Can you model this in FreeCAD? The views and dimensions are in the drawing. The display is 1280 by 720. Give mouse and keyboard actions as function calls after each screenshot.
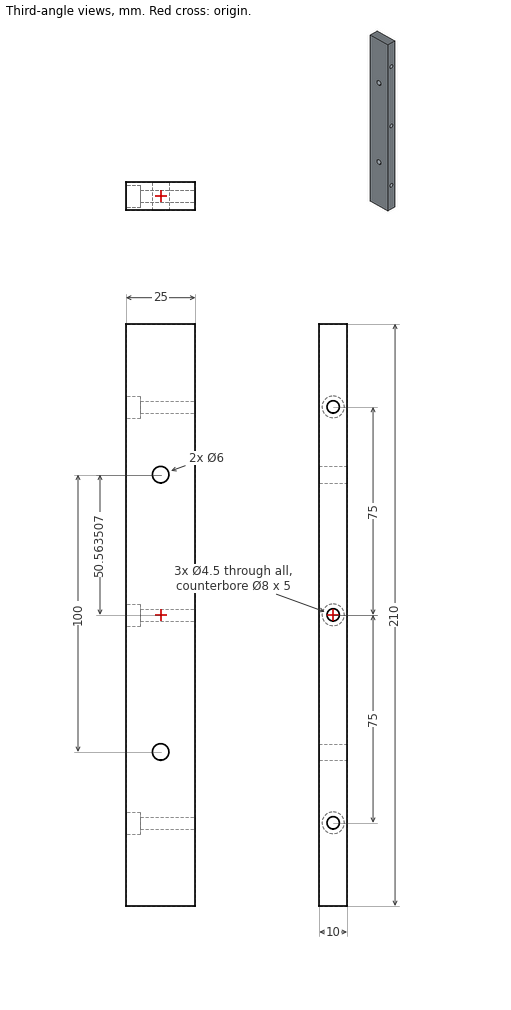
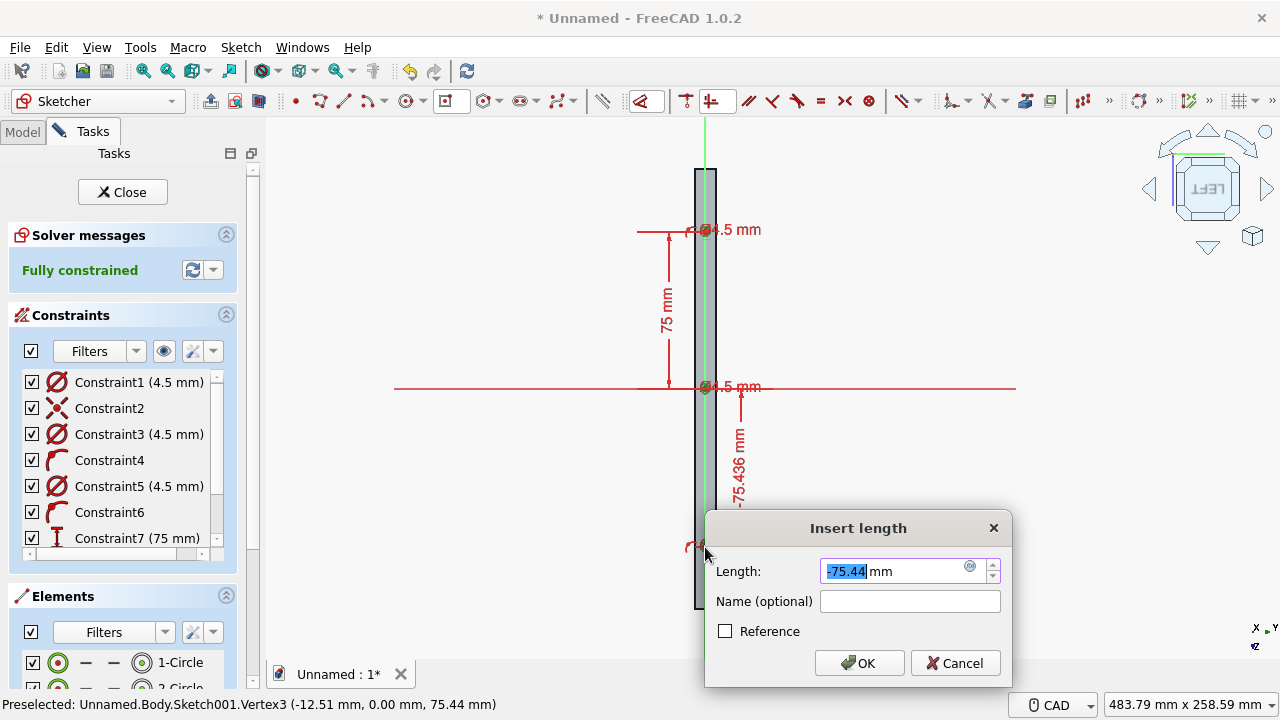
text(-75)
key(Return)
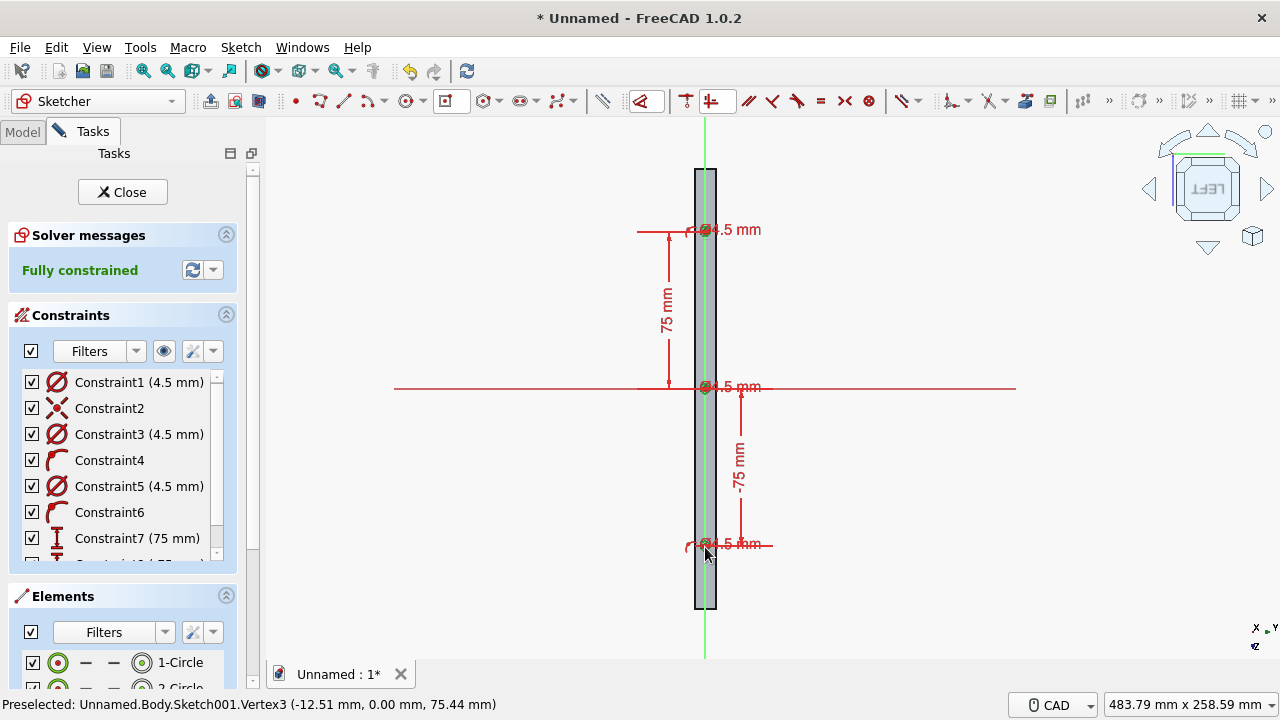
click(123, 192)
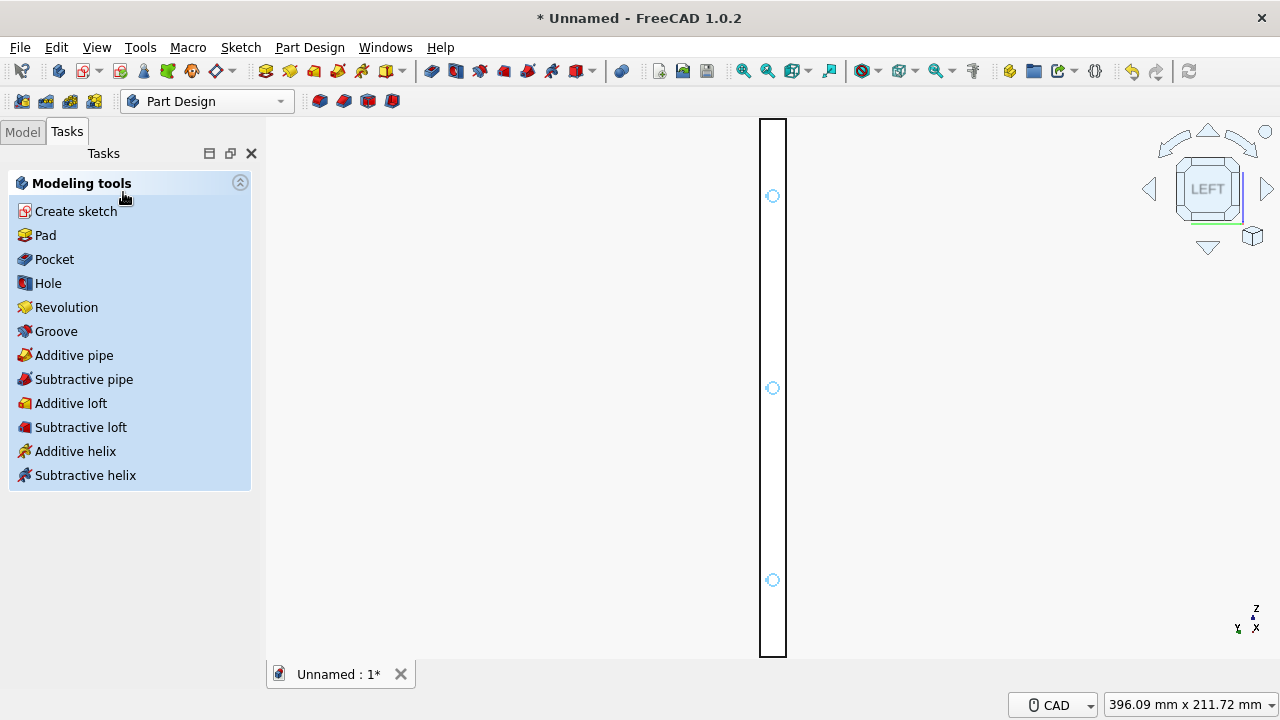
click(456, 72)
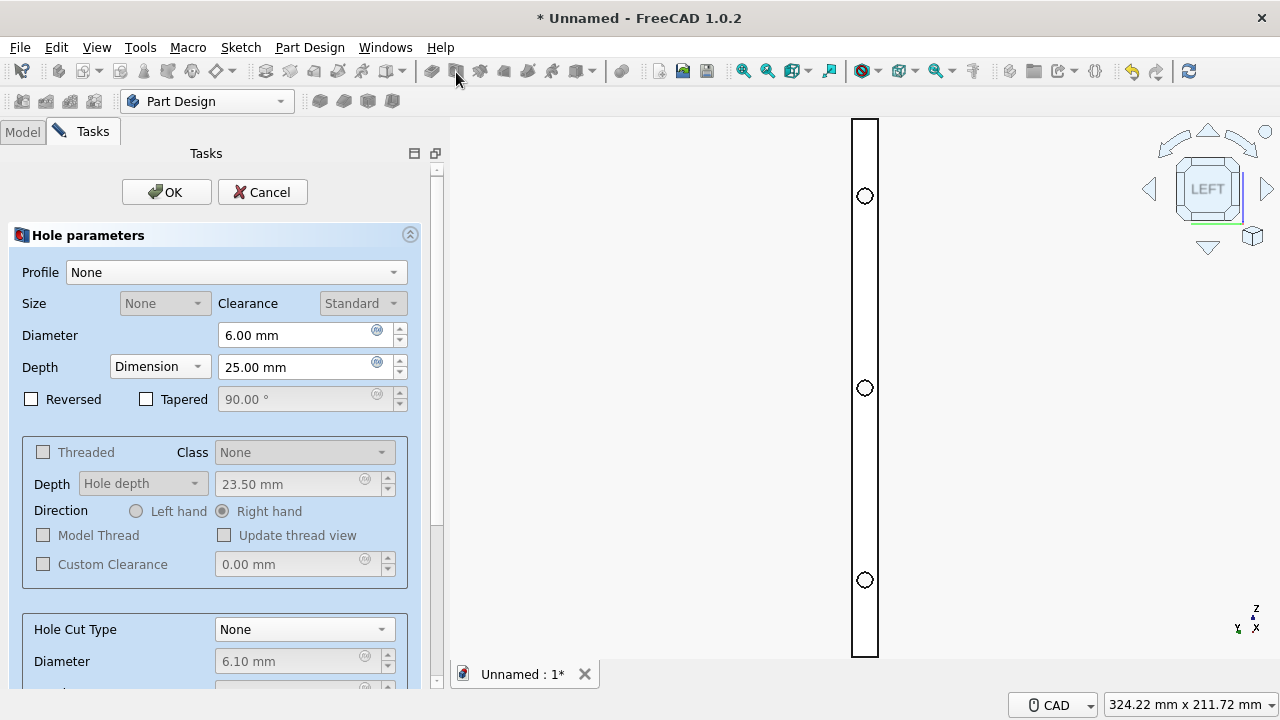
triple_click(305, 335)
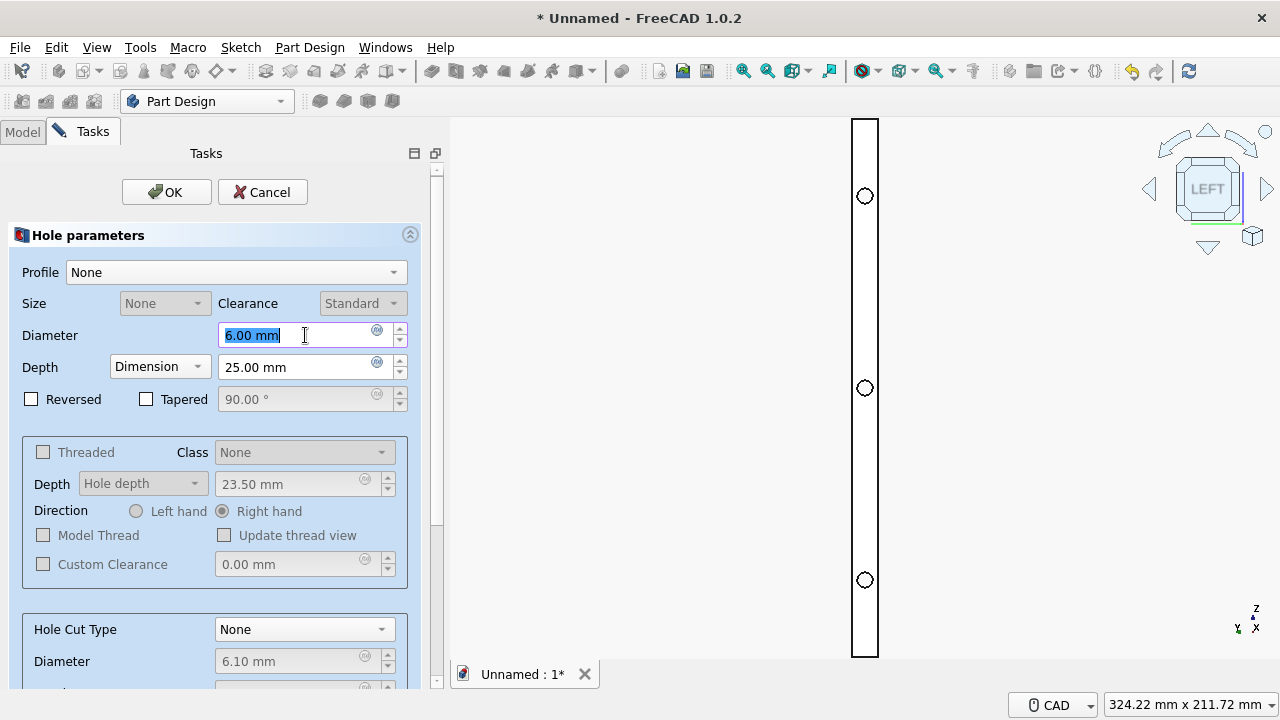
text(4.5)
key(Tab)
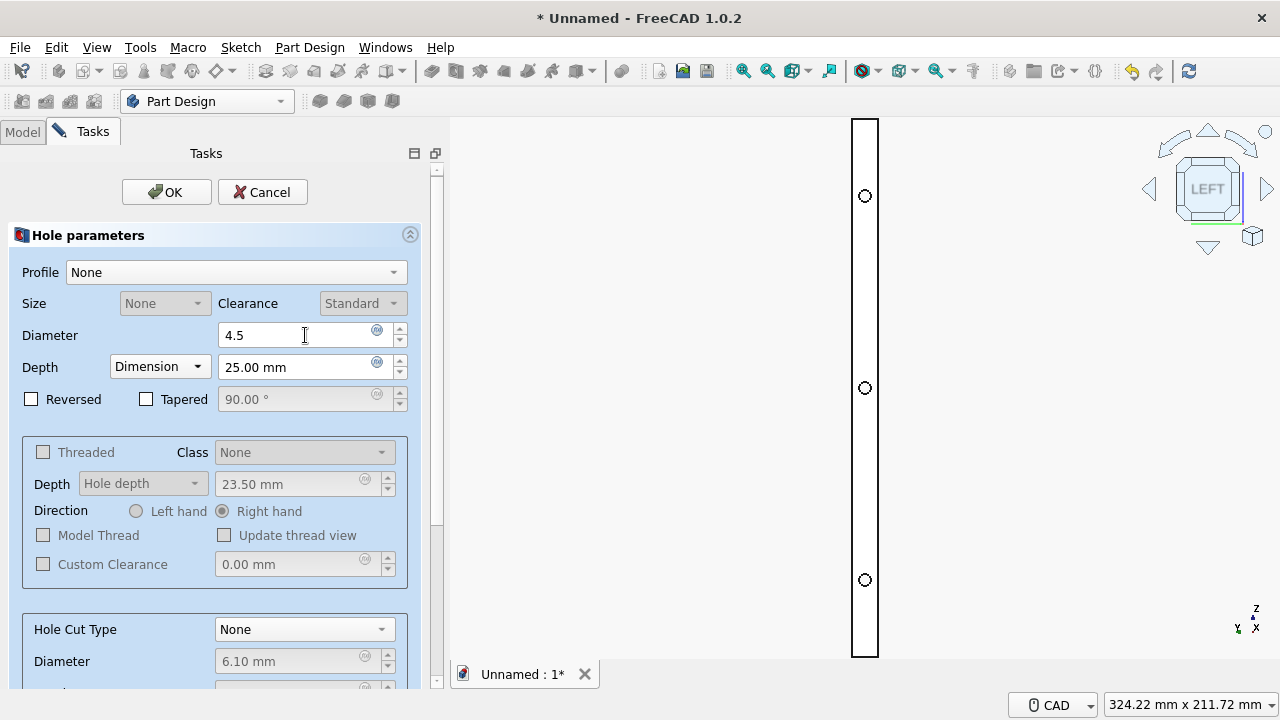
click(161, 366)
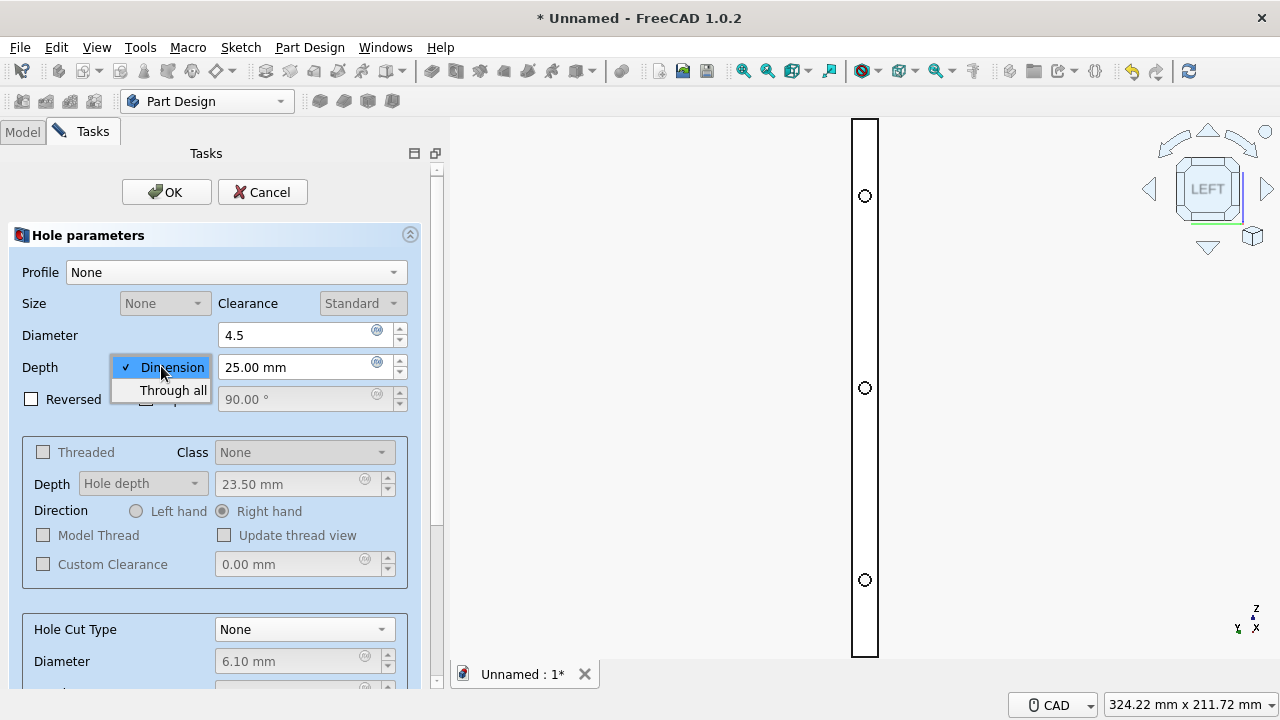
click(160, 390)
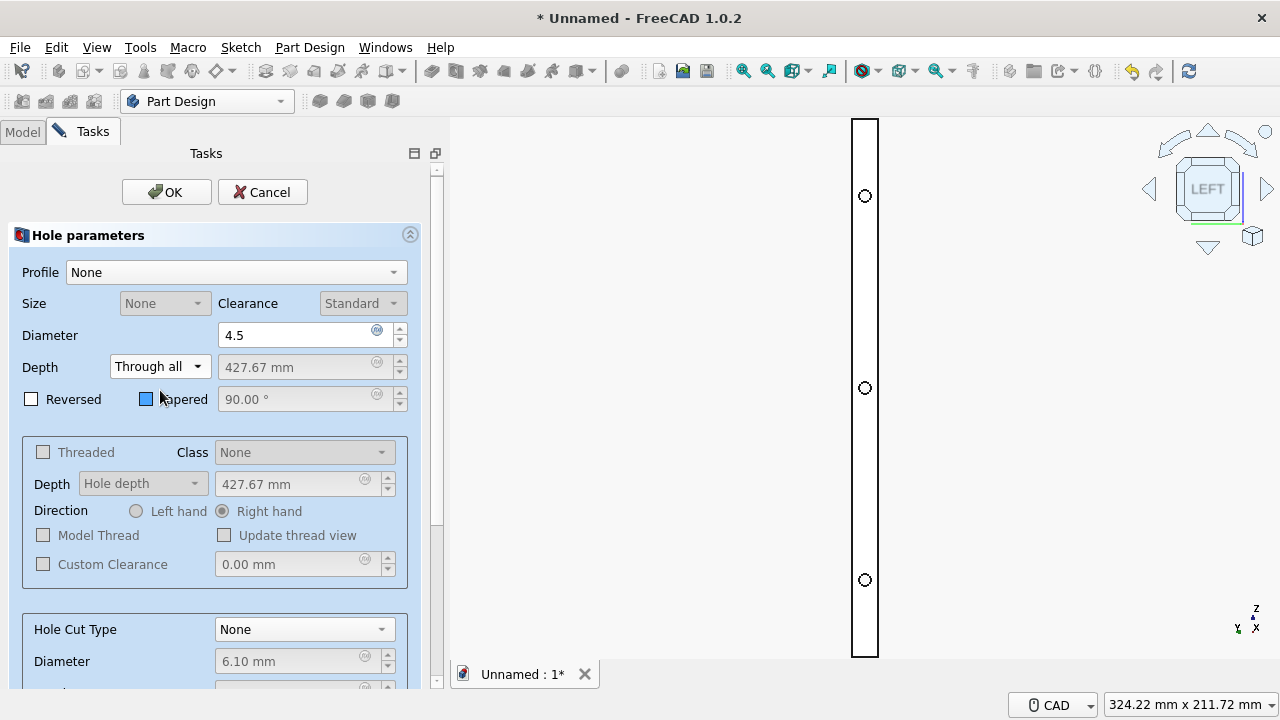
click(306, 630)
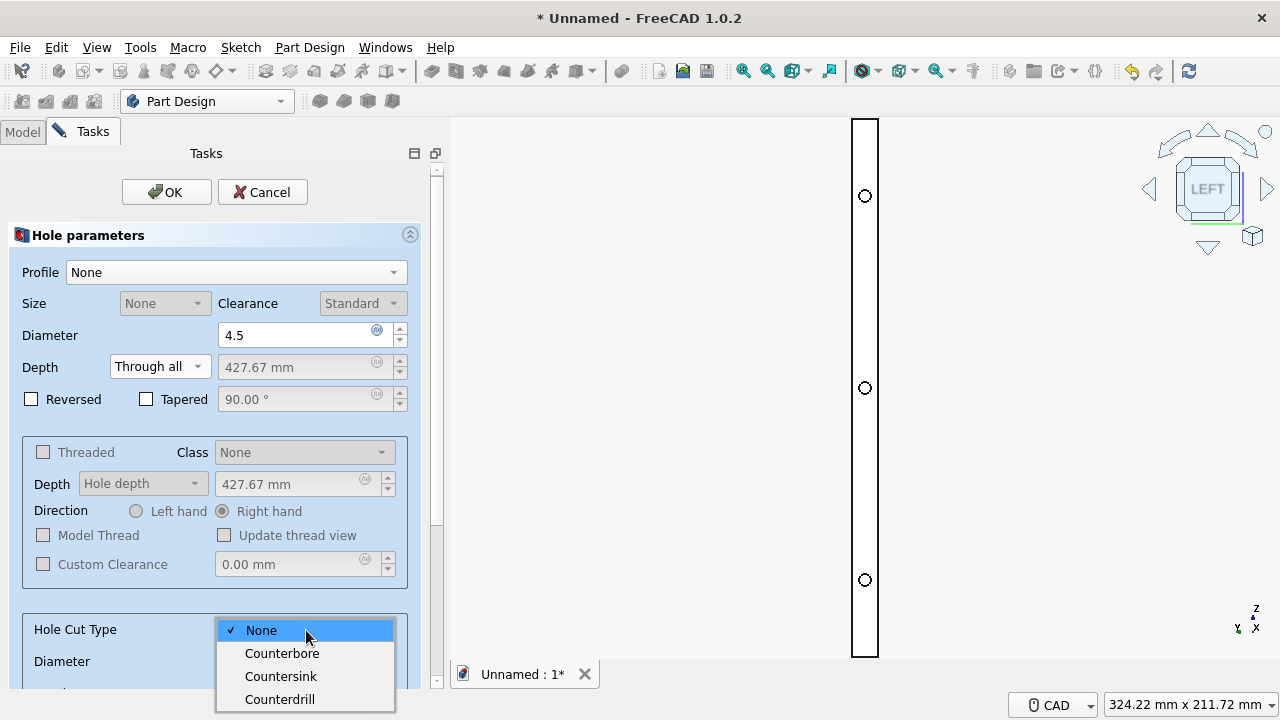
click(304, 654)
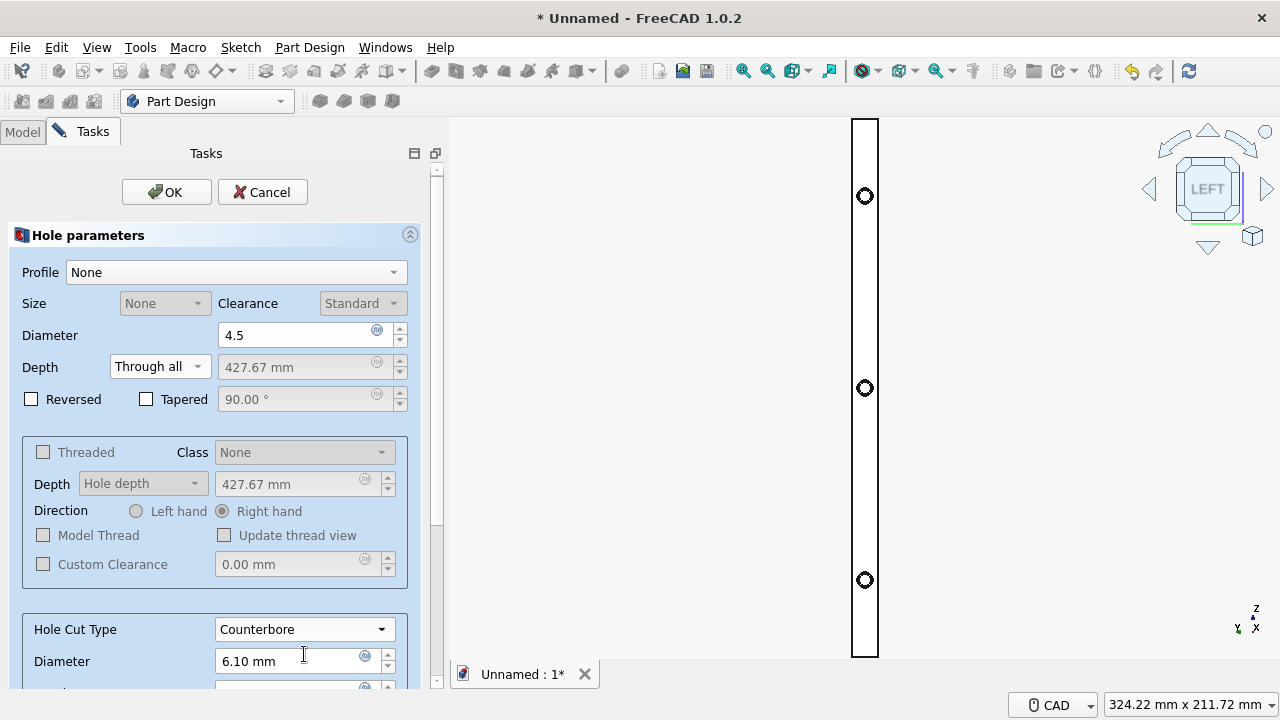
triple_click(298, 661)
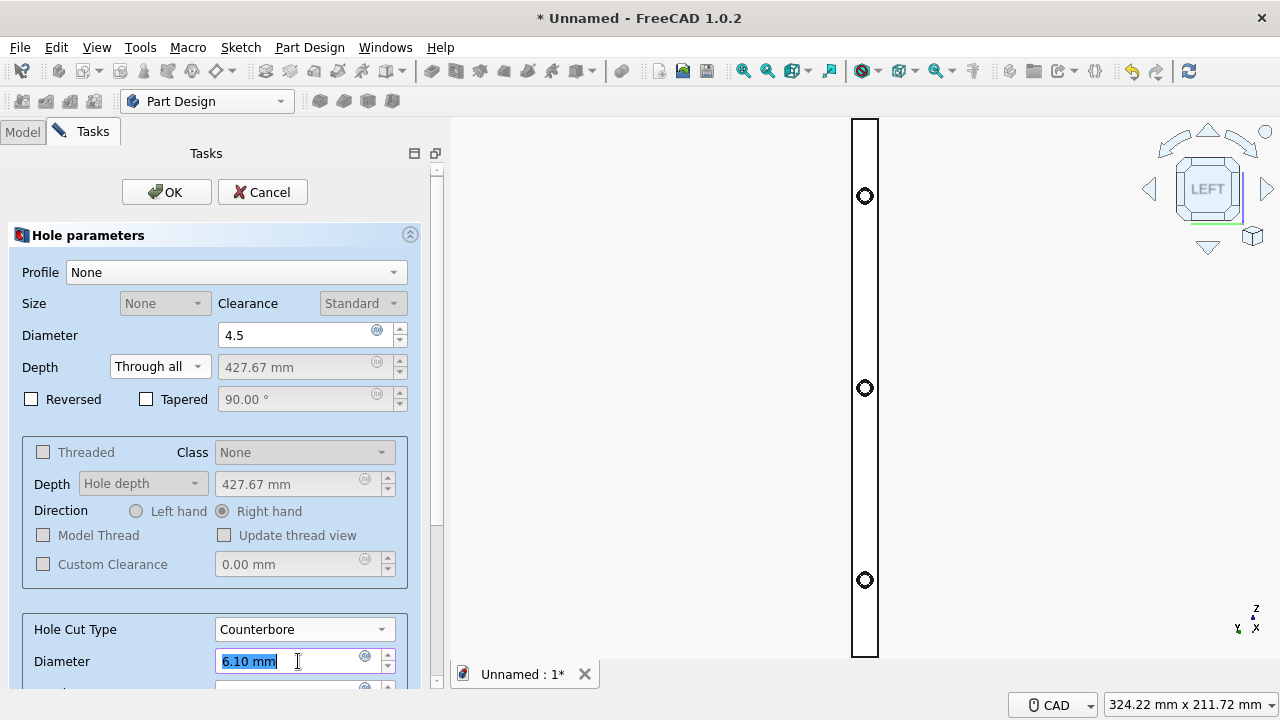
text(8)
key(Tab)